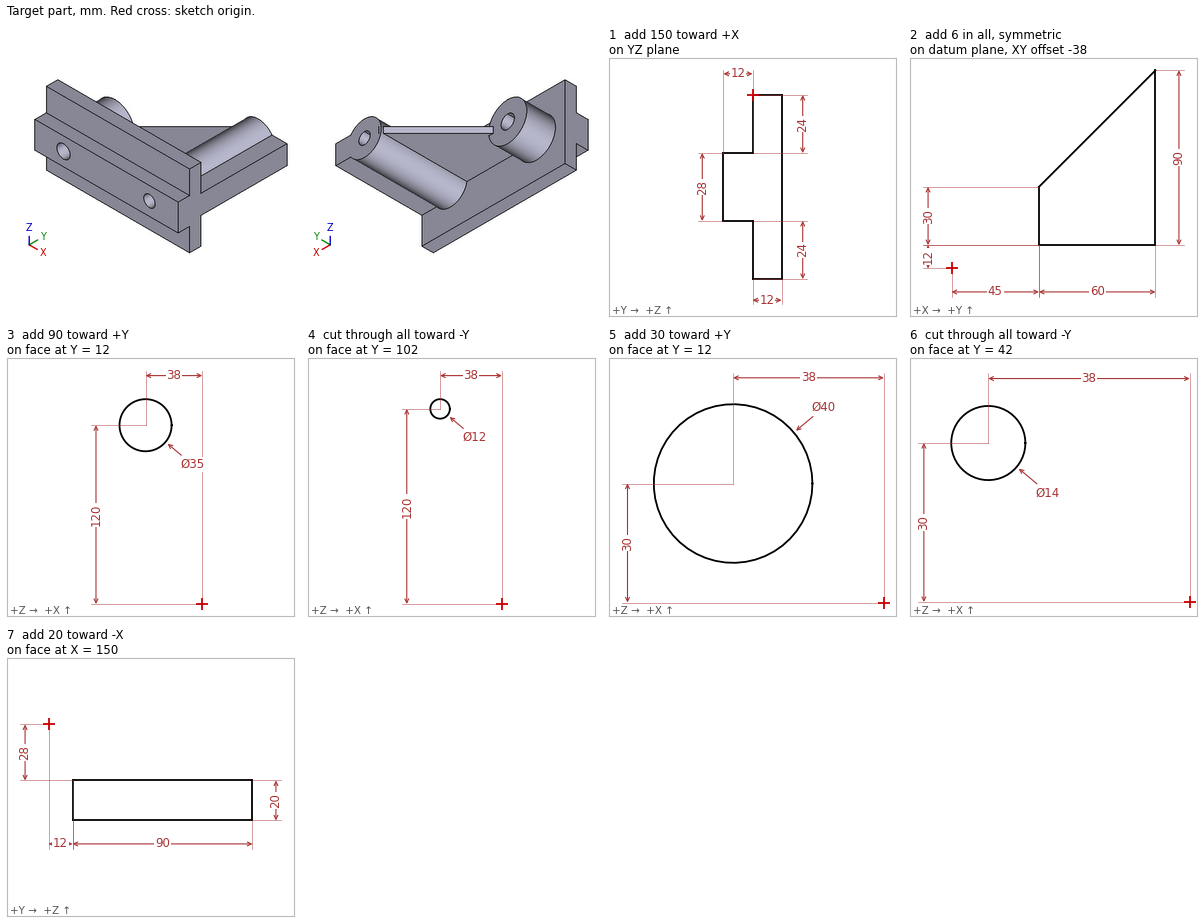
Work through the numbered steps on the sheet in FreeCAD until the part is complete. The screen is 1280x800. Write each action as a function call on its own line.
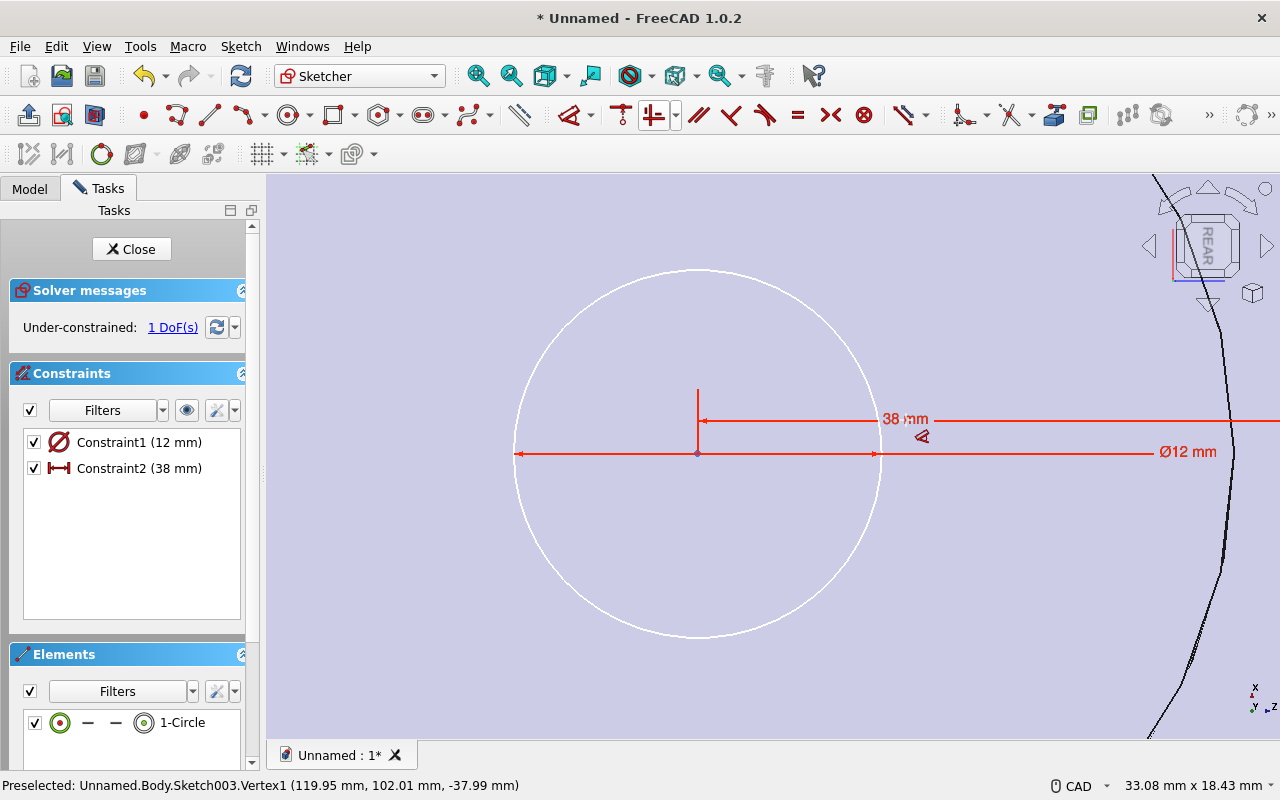
click(698, 454)
click(664, 582)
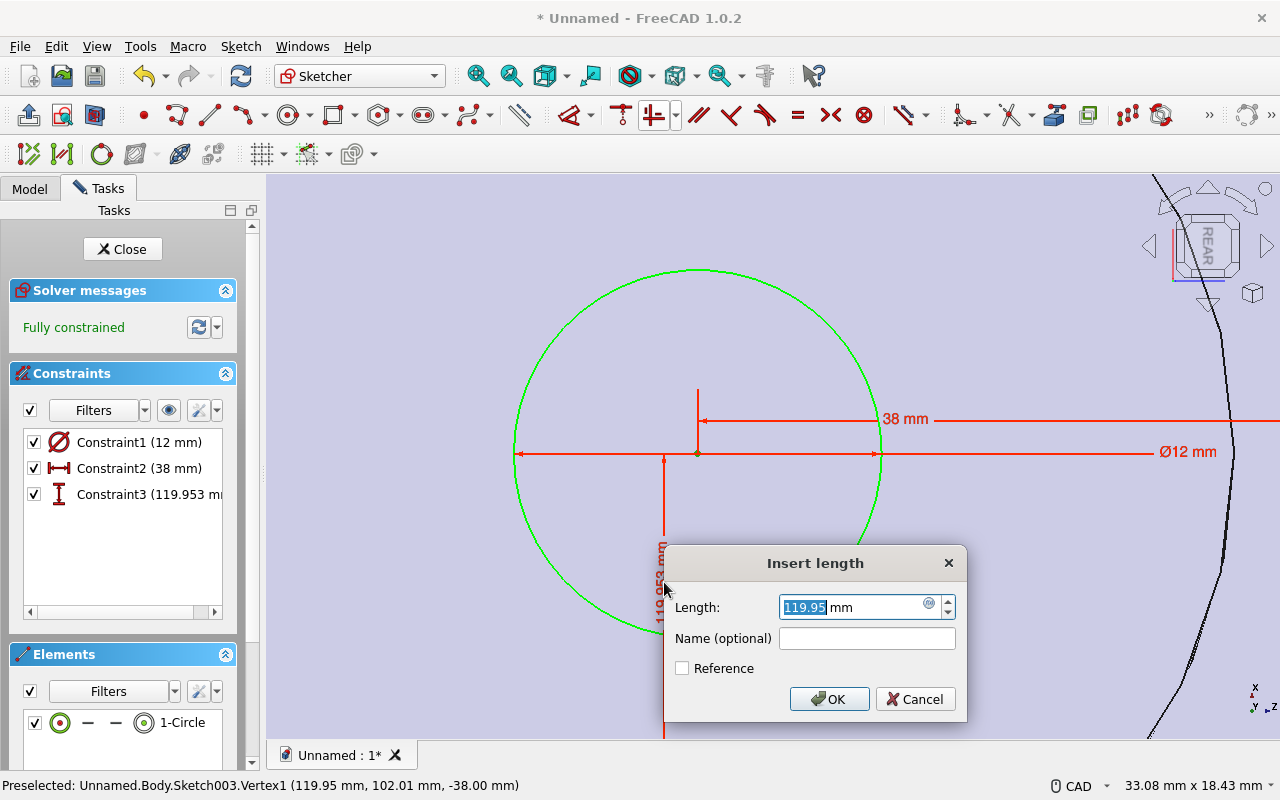
text(120)
key(Return)
key(Escape)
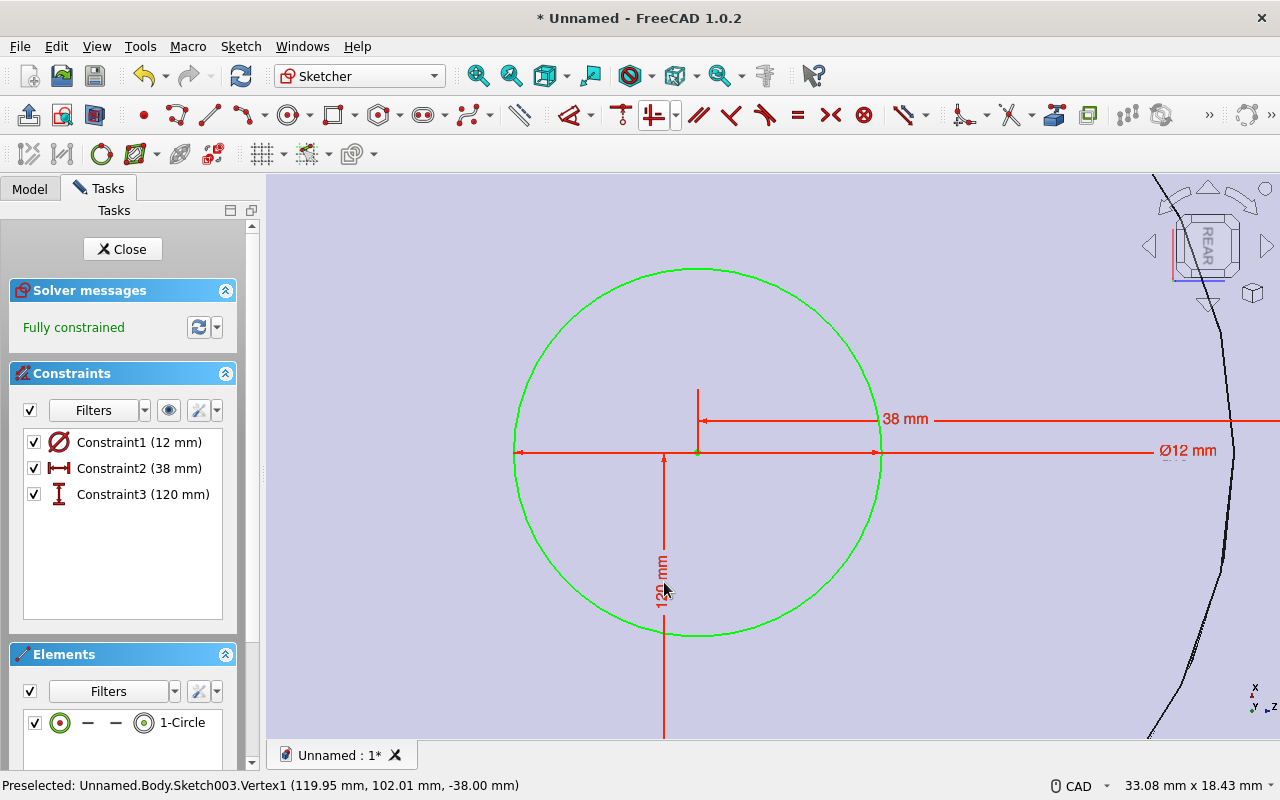
click(123, 249)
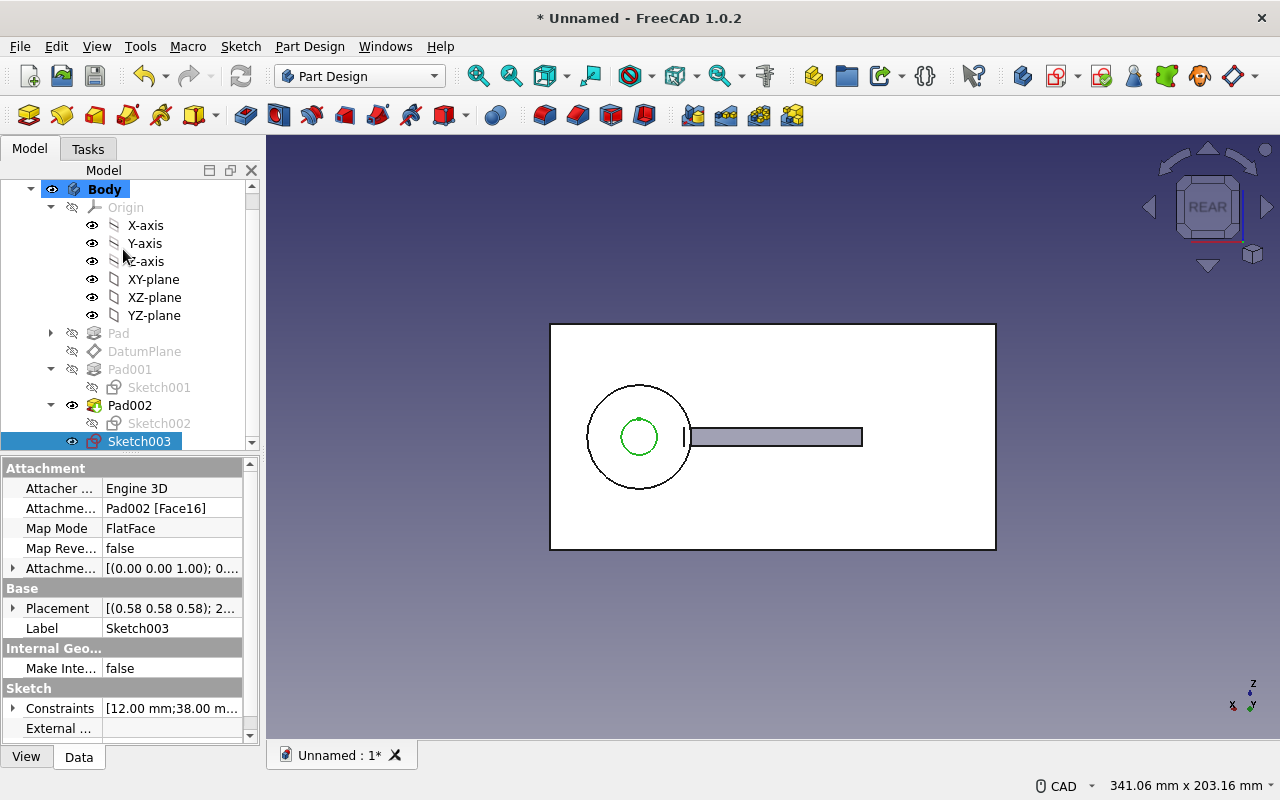
click(246, 116)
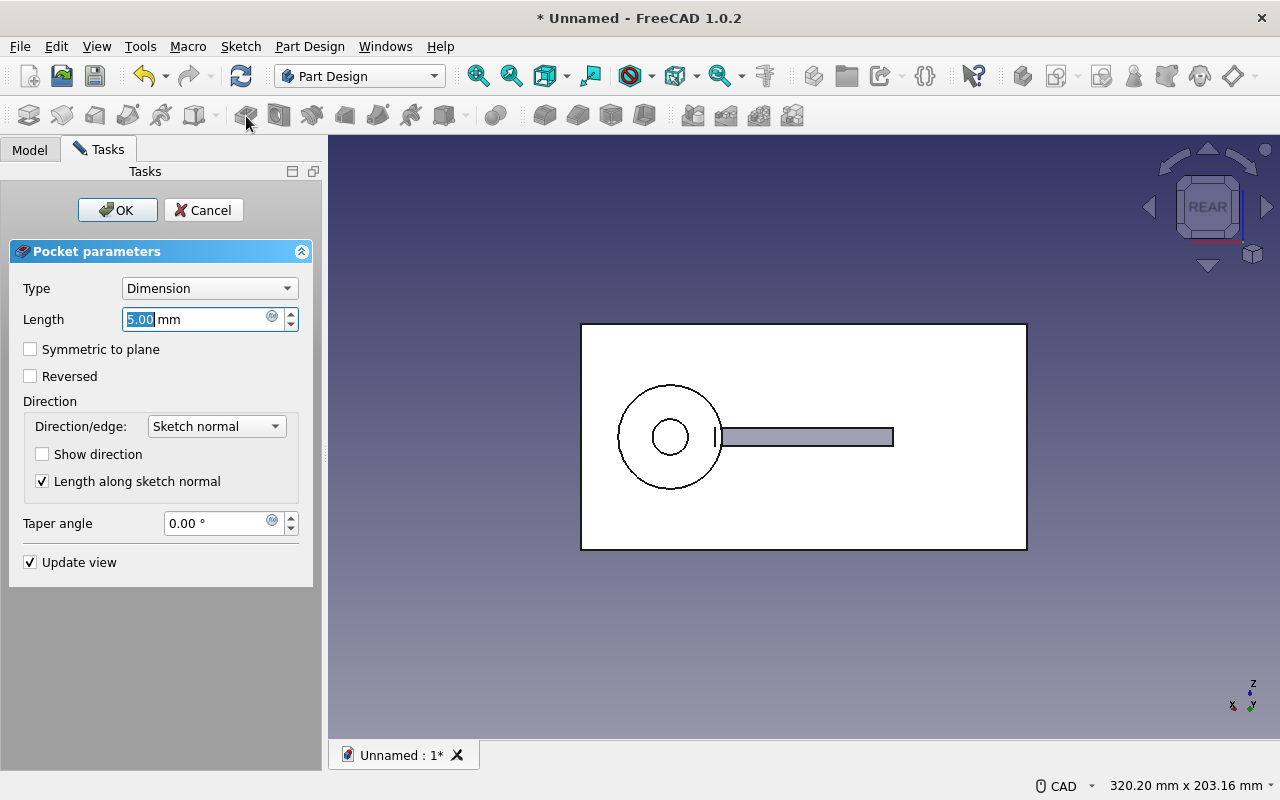
click(210, 288)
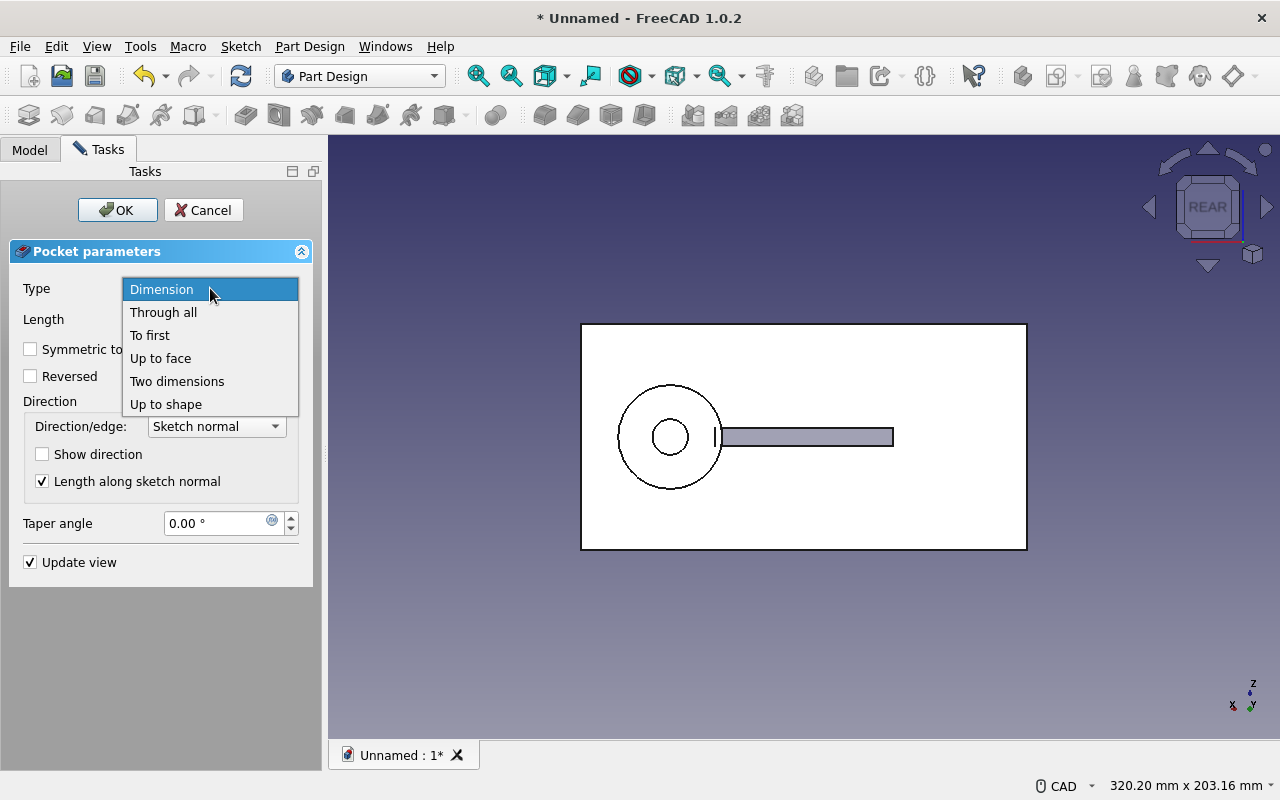
click(208, 312)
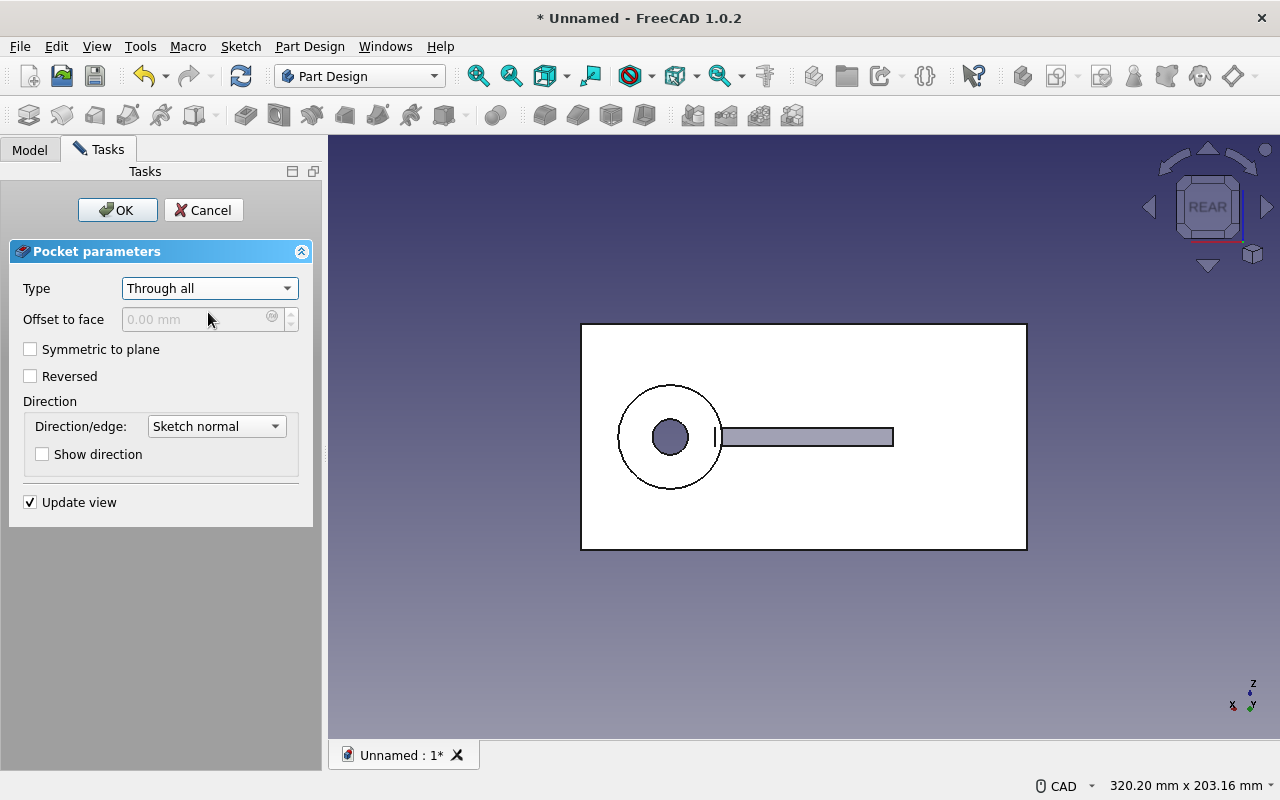
click(118, 210)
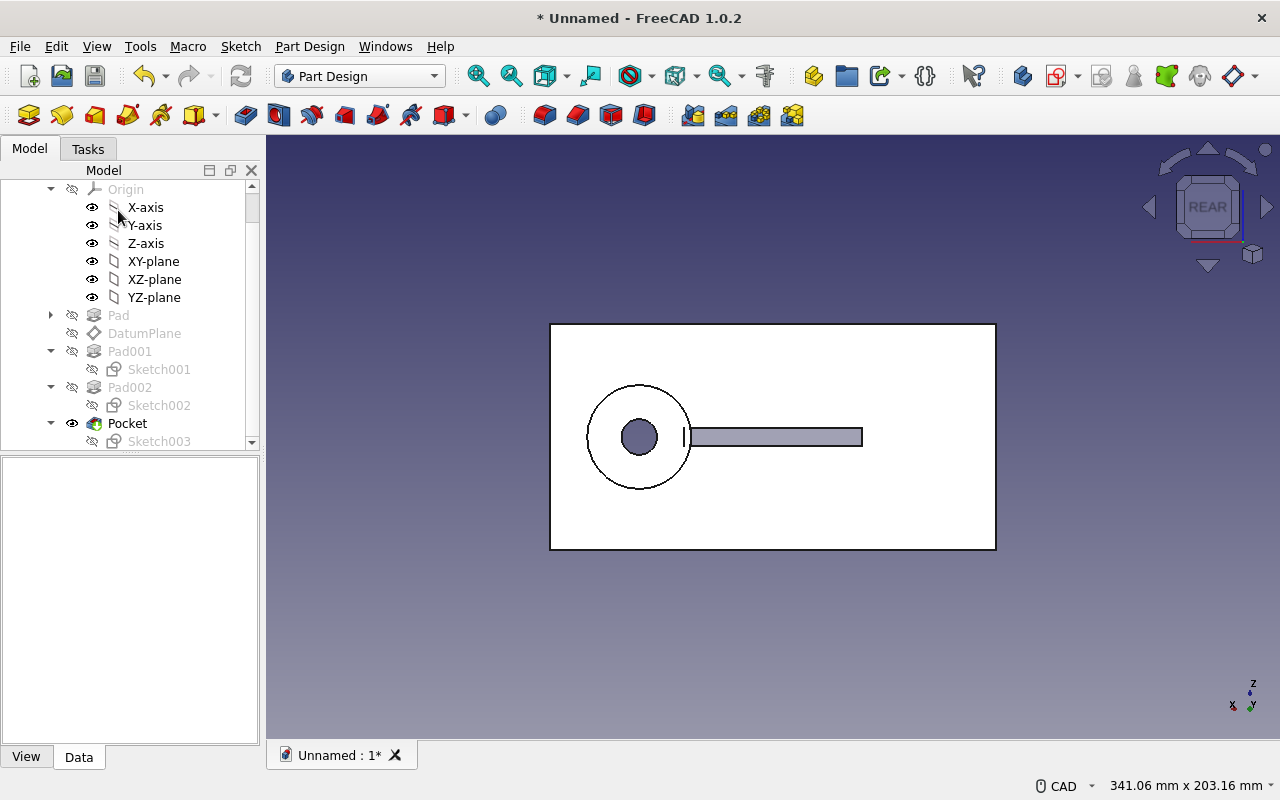
click(479, 76)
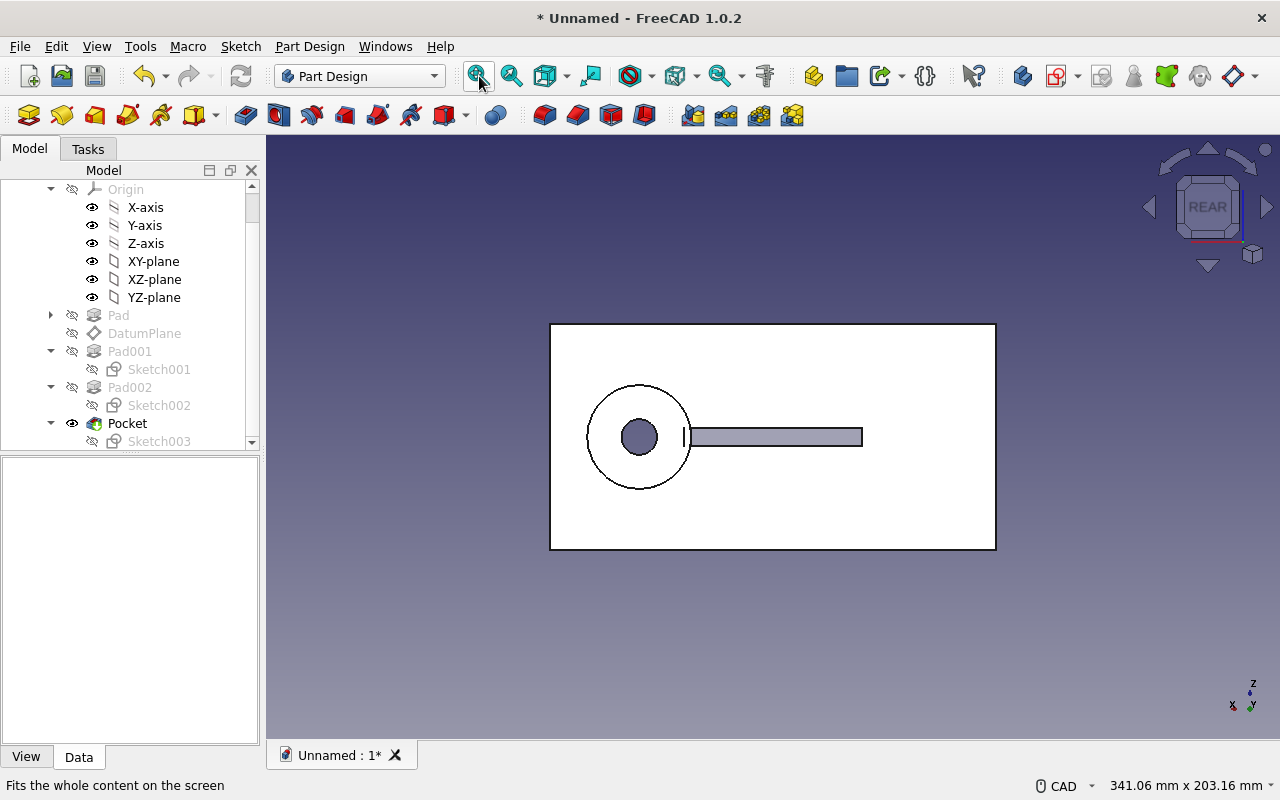
click(900, 371)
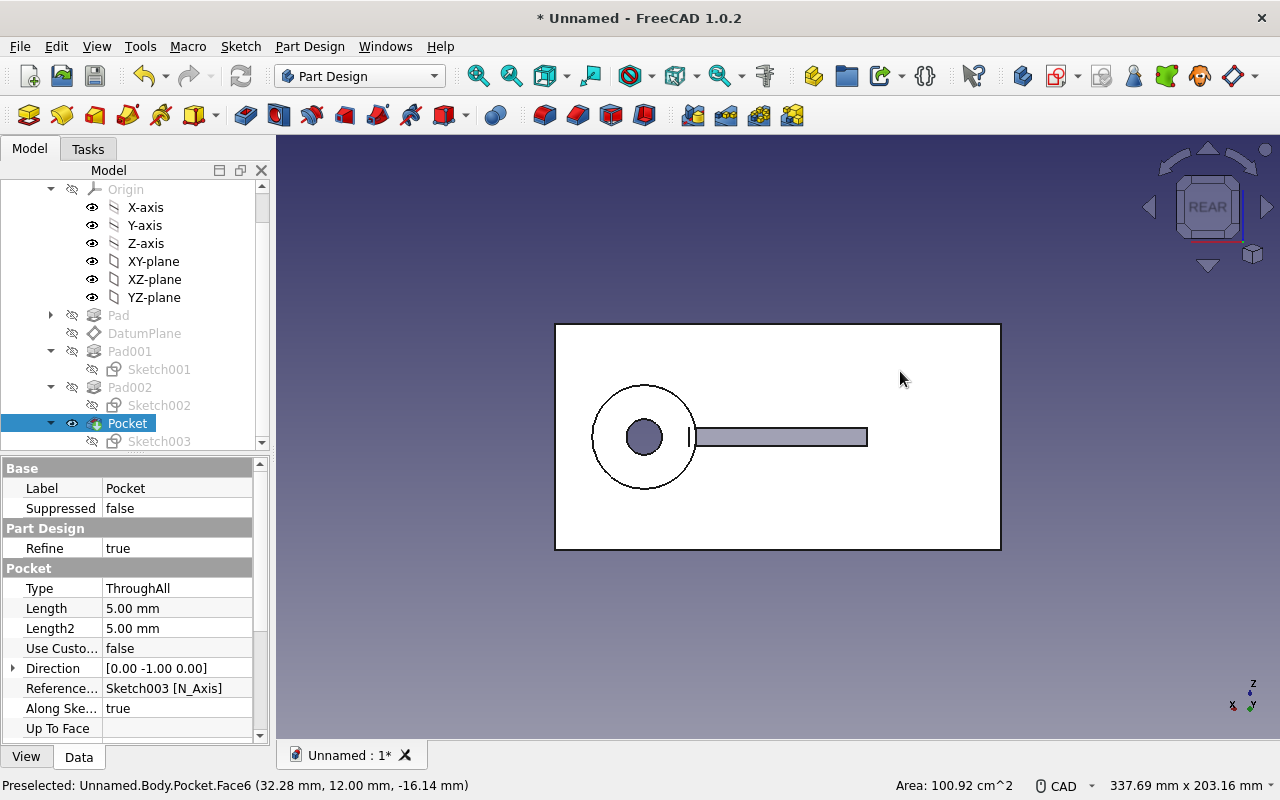
click(1056, 76)